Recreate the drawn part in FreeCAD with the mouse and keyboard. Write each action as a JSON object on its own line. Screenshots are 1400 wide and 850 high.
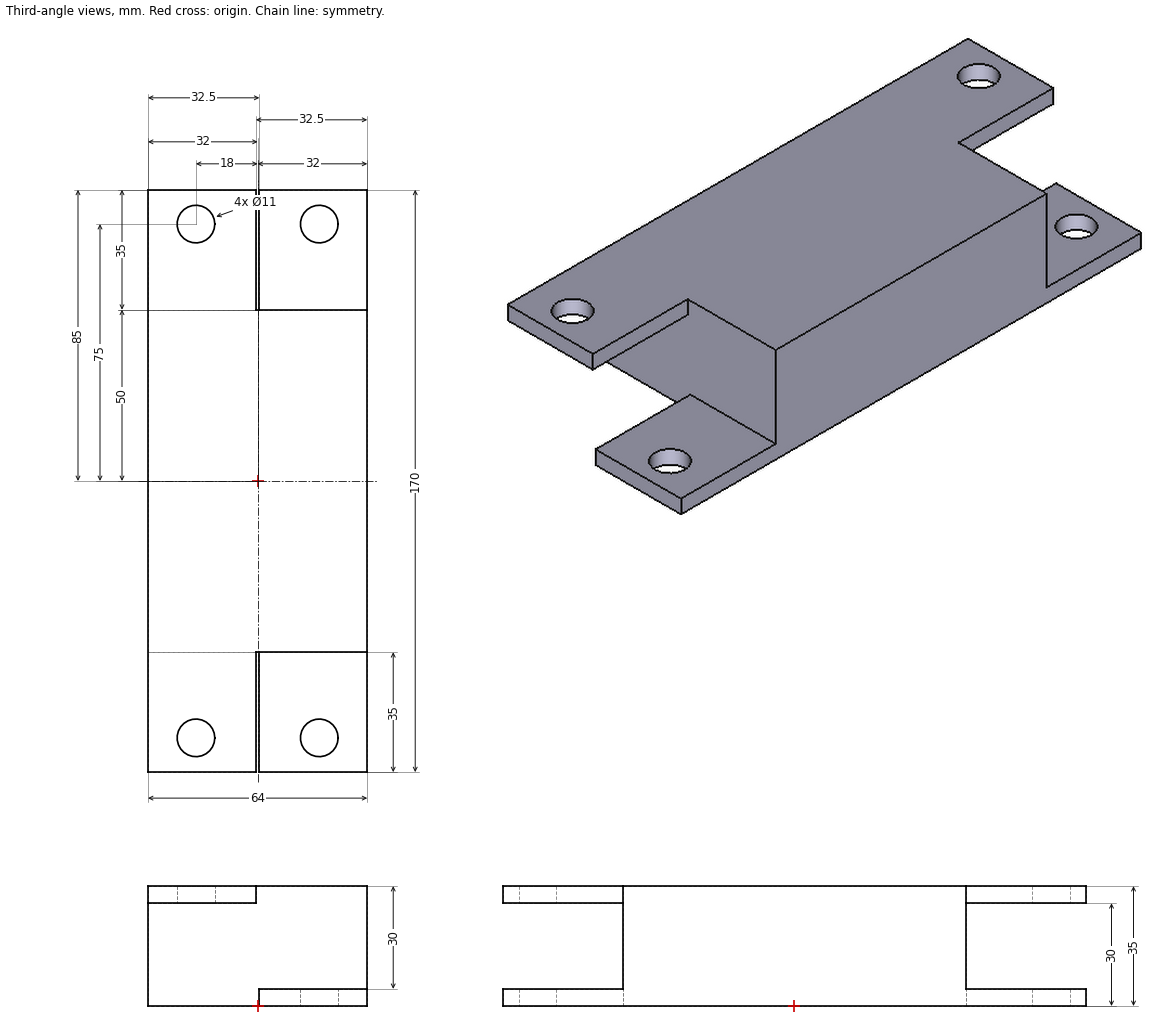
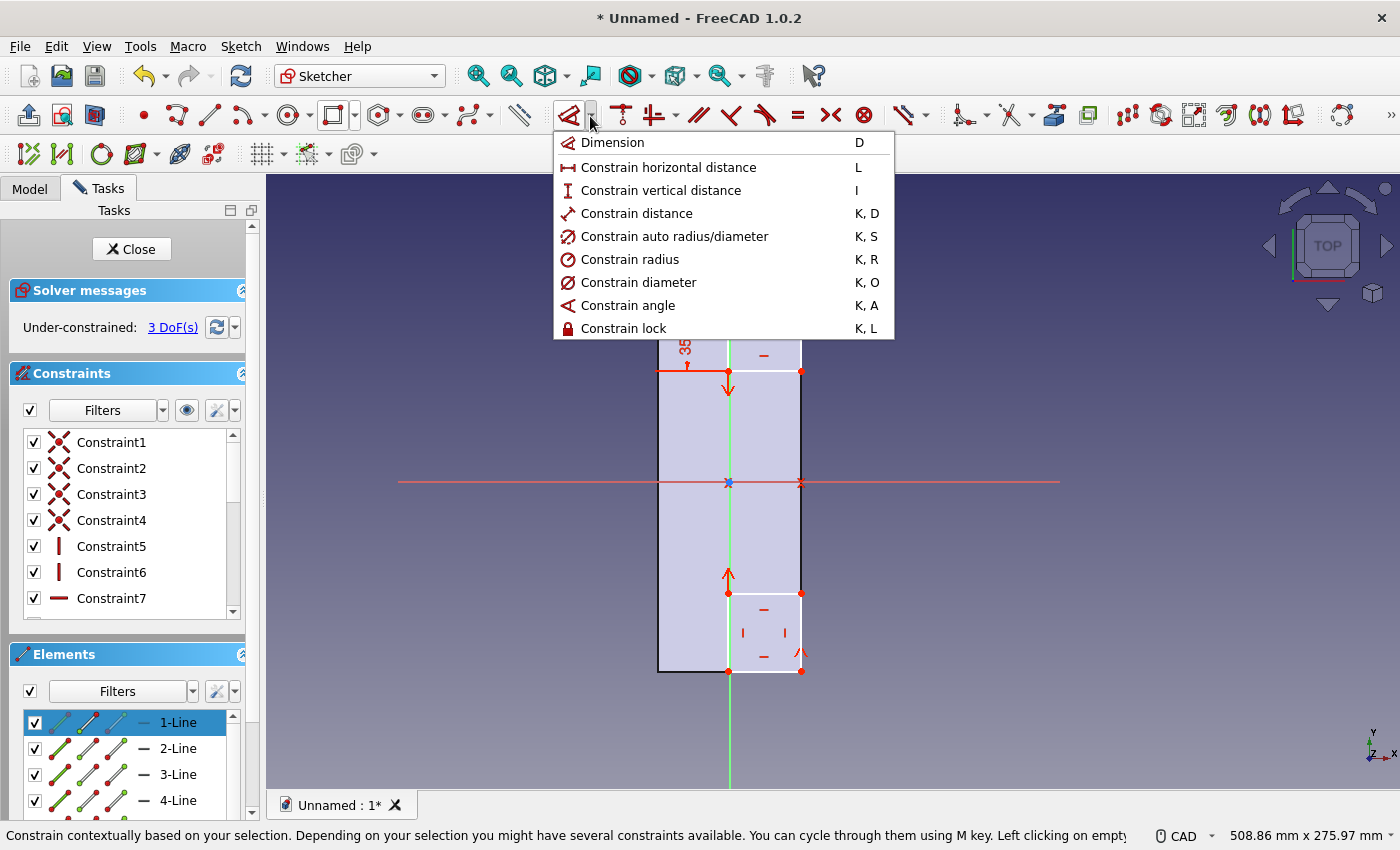
{"action": "left_click", "coordinate": [724, 190]}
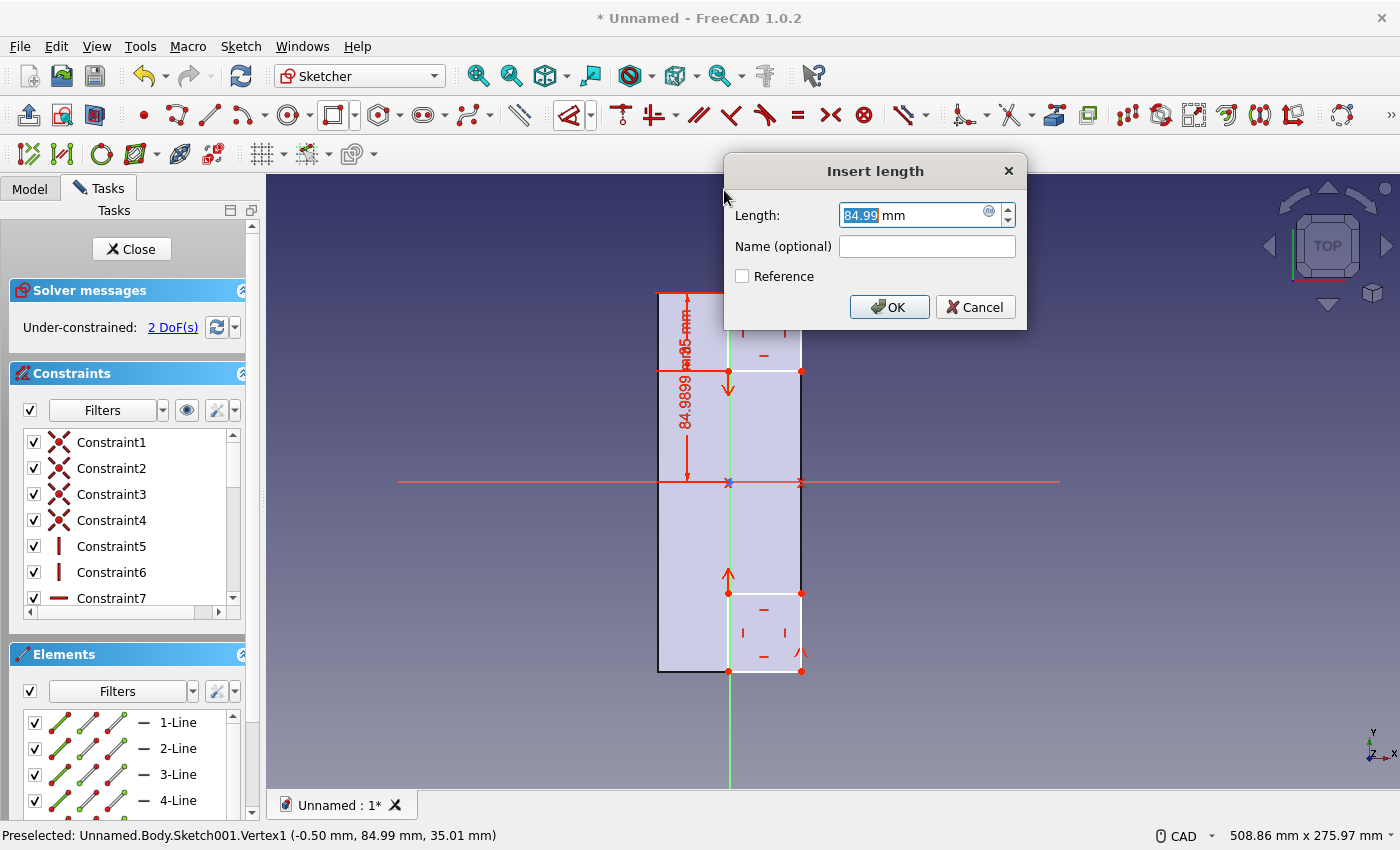
{"action": "type", "text": "85"}
{"action": "key", "text": "Return"}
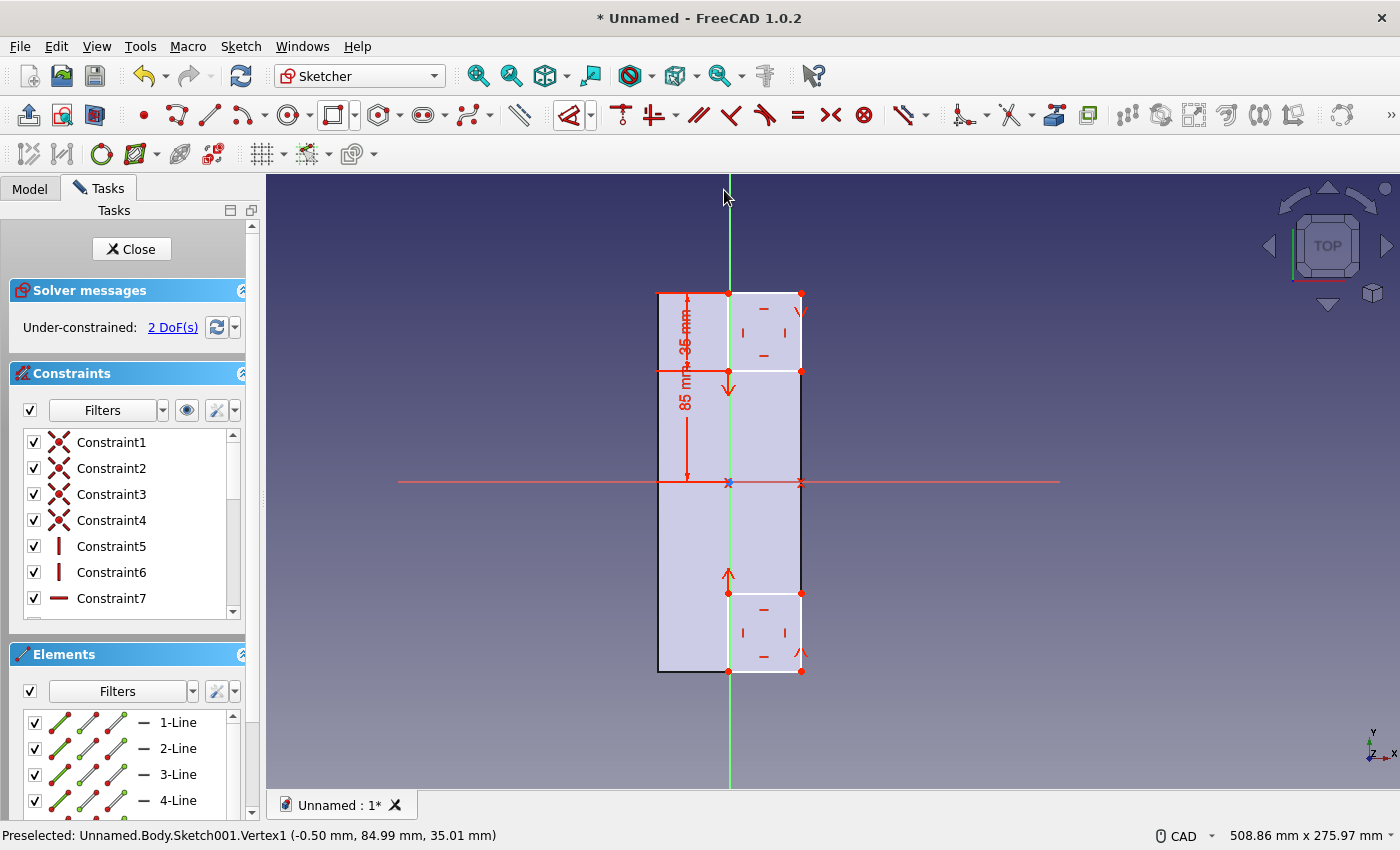
{"action": "left_click", "coordinate": [801, 371]}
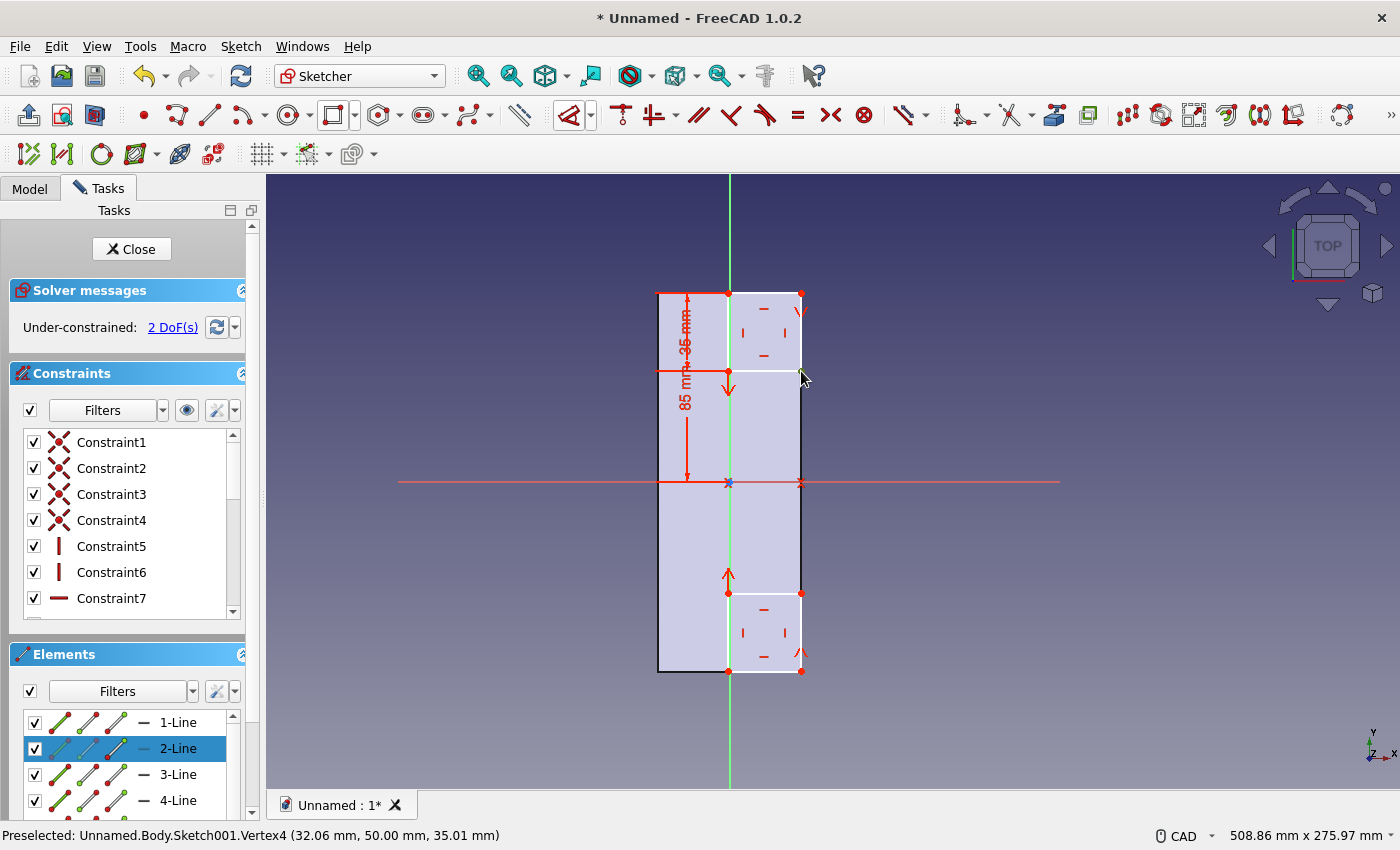
{"action": "left_click", "coordinate": [590, 116]}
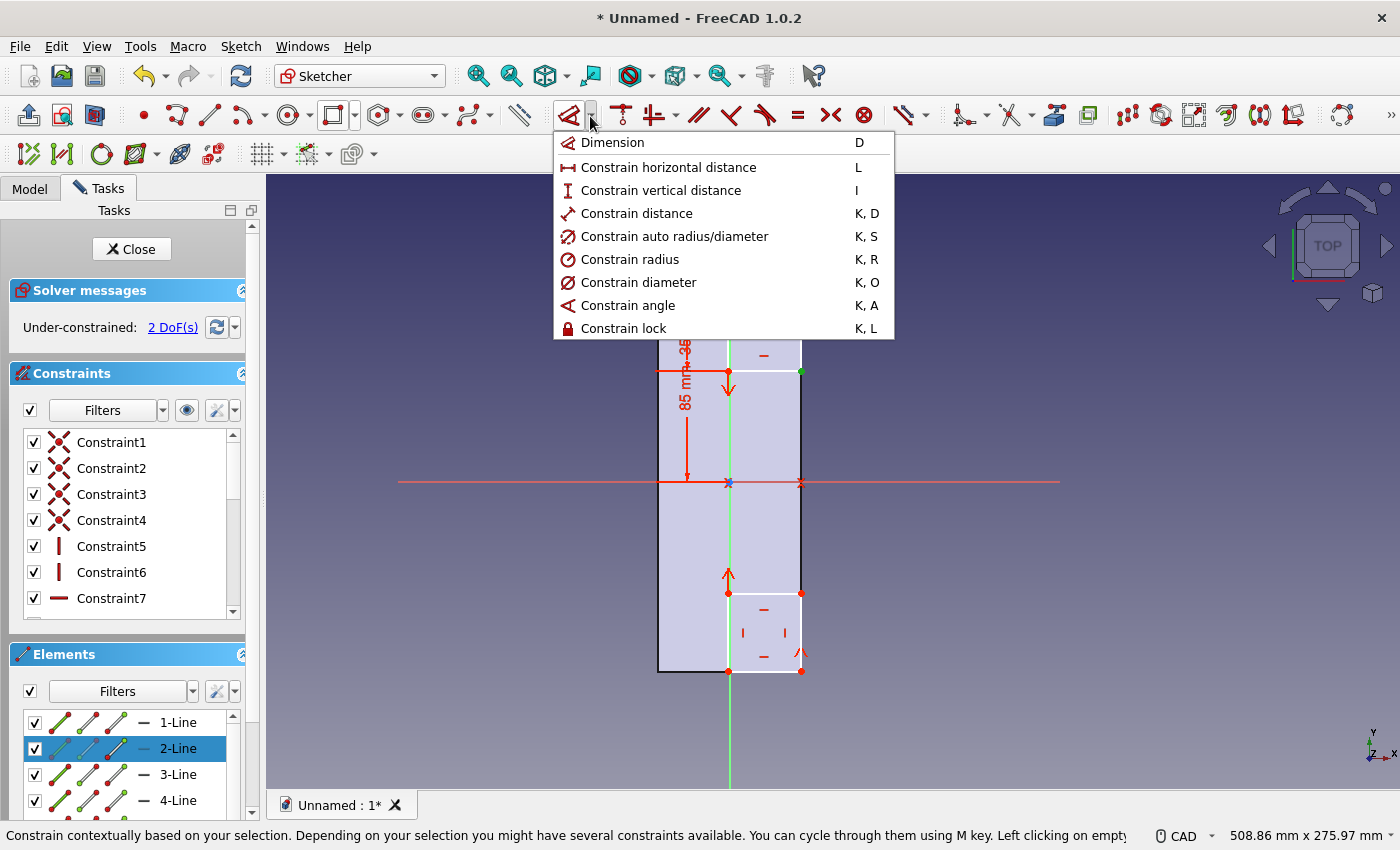
{"action": "left_click", "coordinate": [724, 168]}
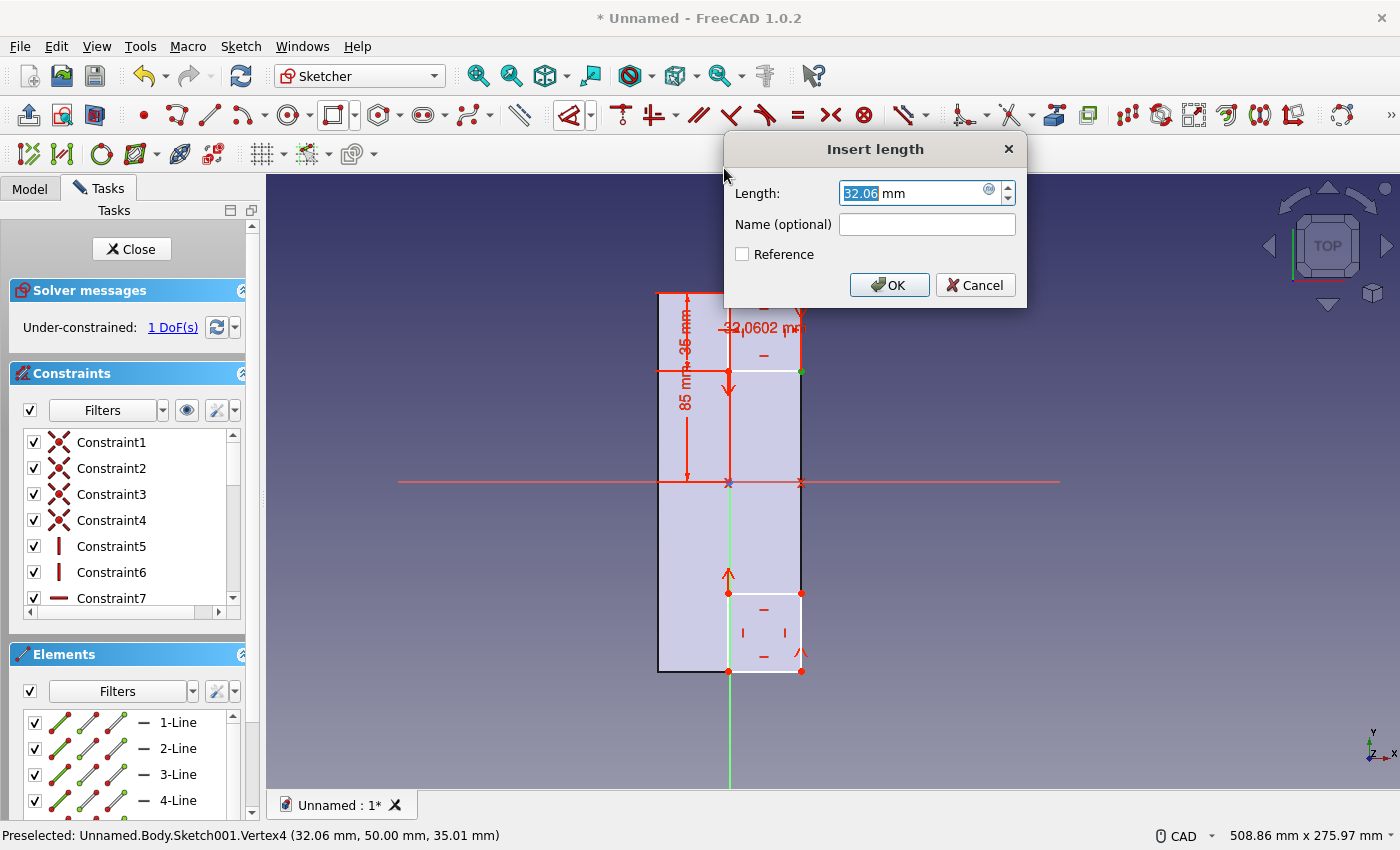
{"action": "type", "text": "32"}
{"action": "key", "text": "Return"}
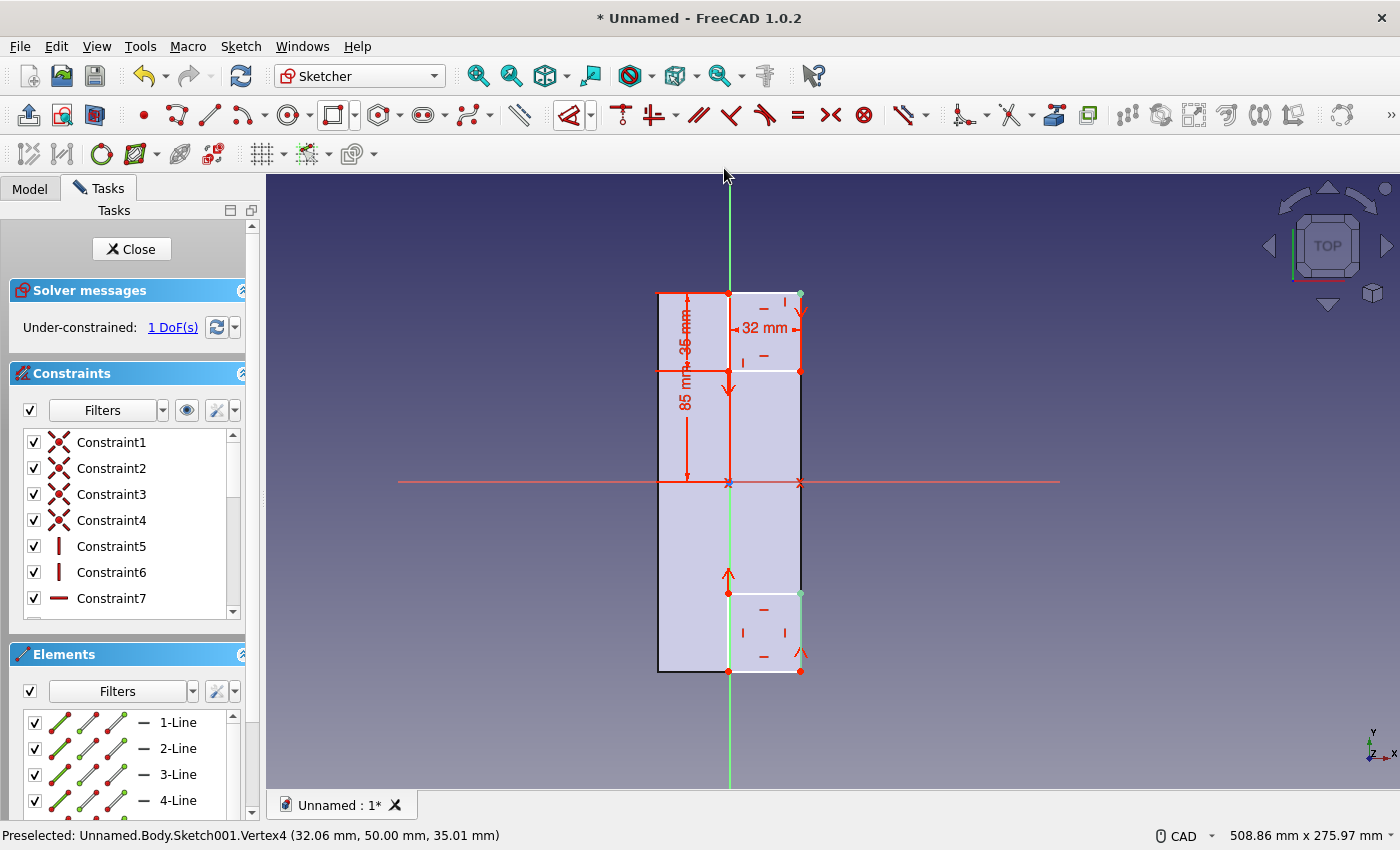
{"action": "left_click", "coordinate": [750, 371]}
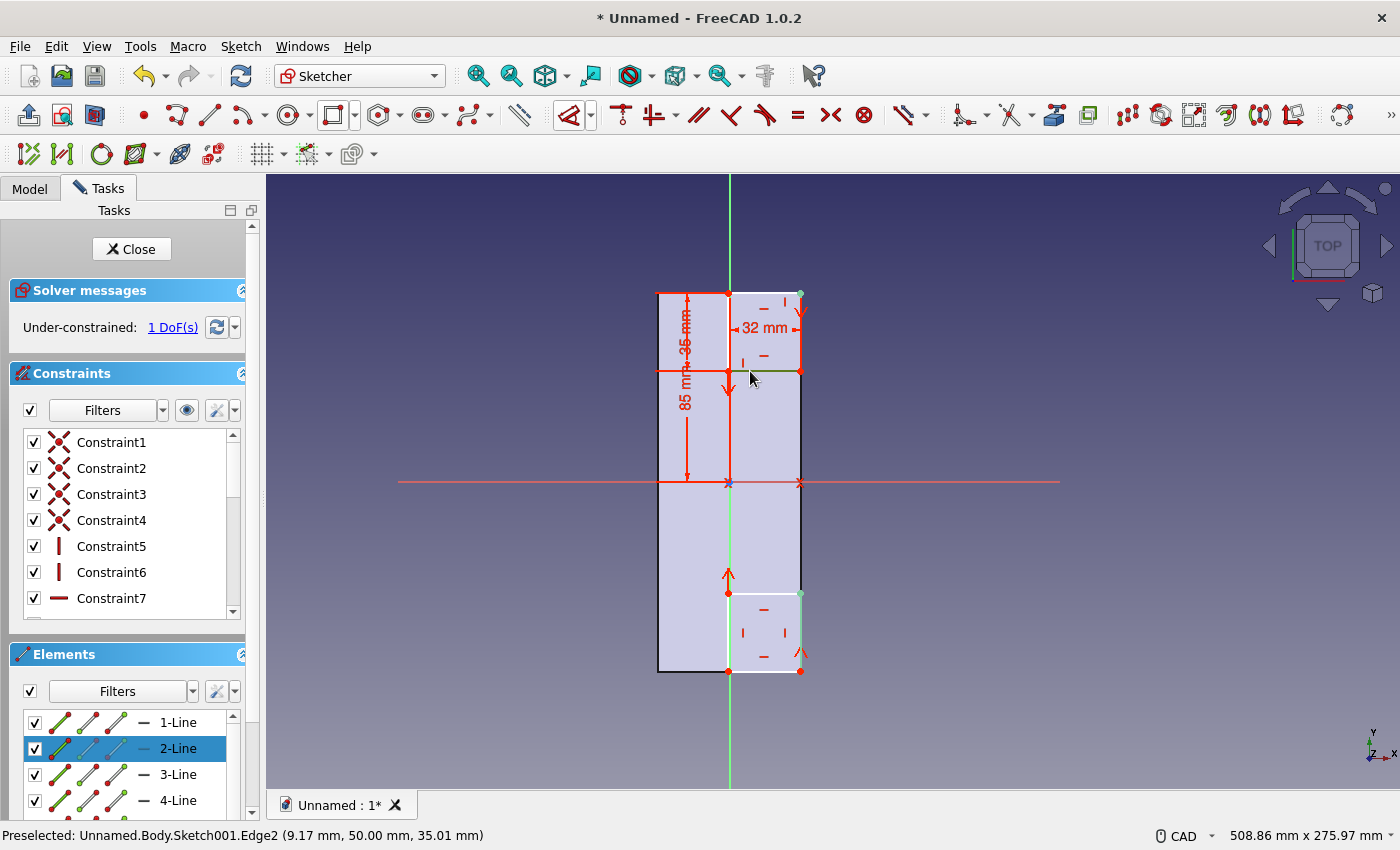
{"action": "left_click", "coordinate": [590, 116]}